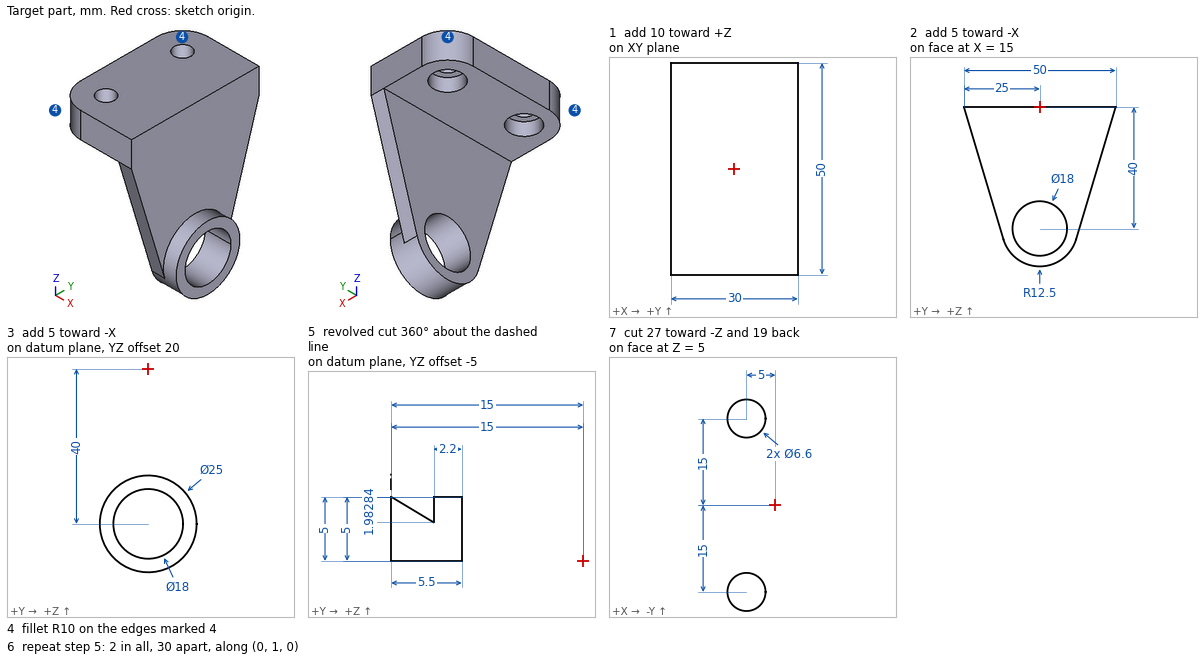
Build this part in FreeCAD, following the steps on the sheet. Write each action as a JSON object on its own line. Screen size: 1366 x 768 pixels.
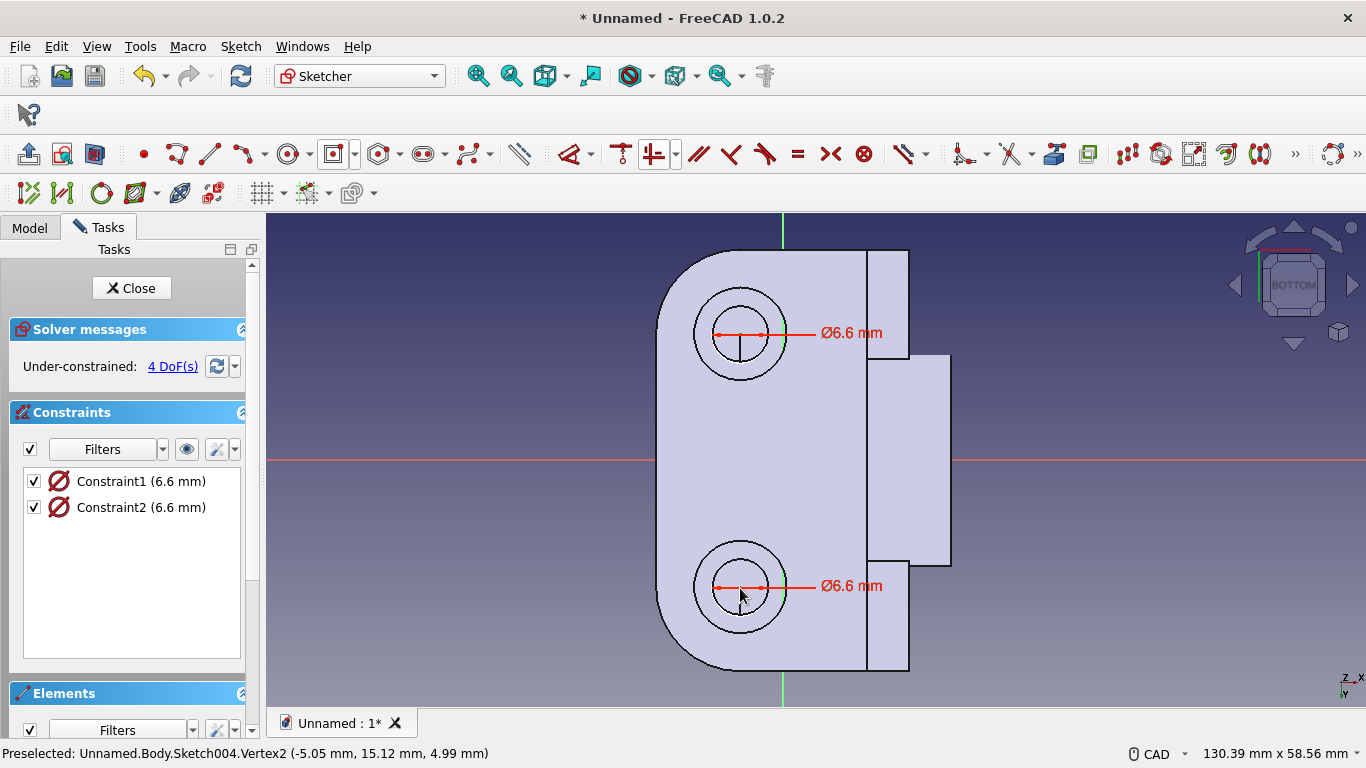
{"action": "key", "text": "v"}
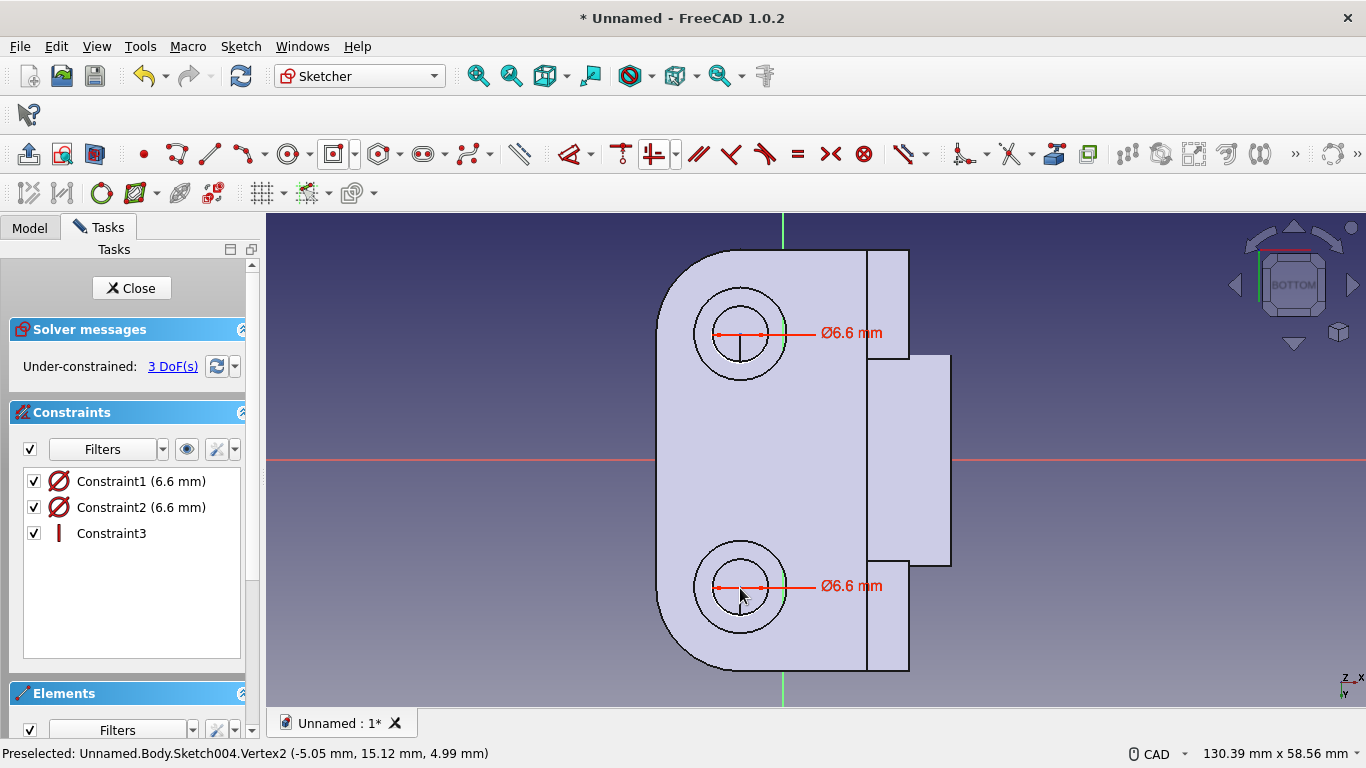
{"action": "left_click", "coordinate": [568, 154]}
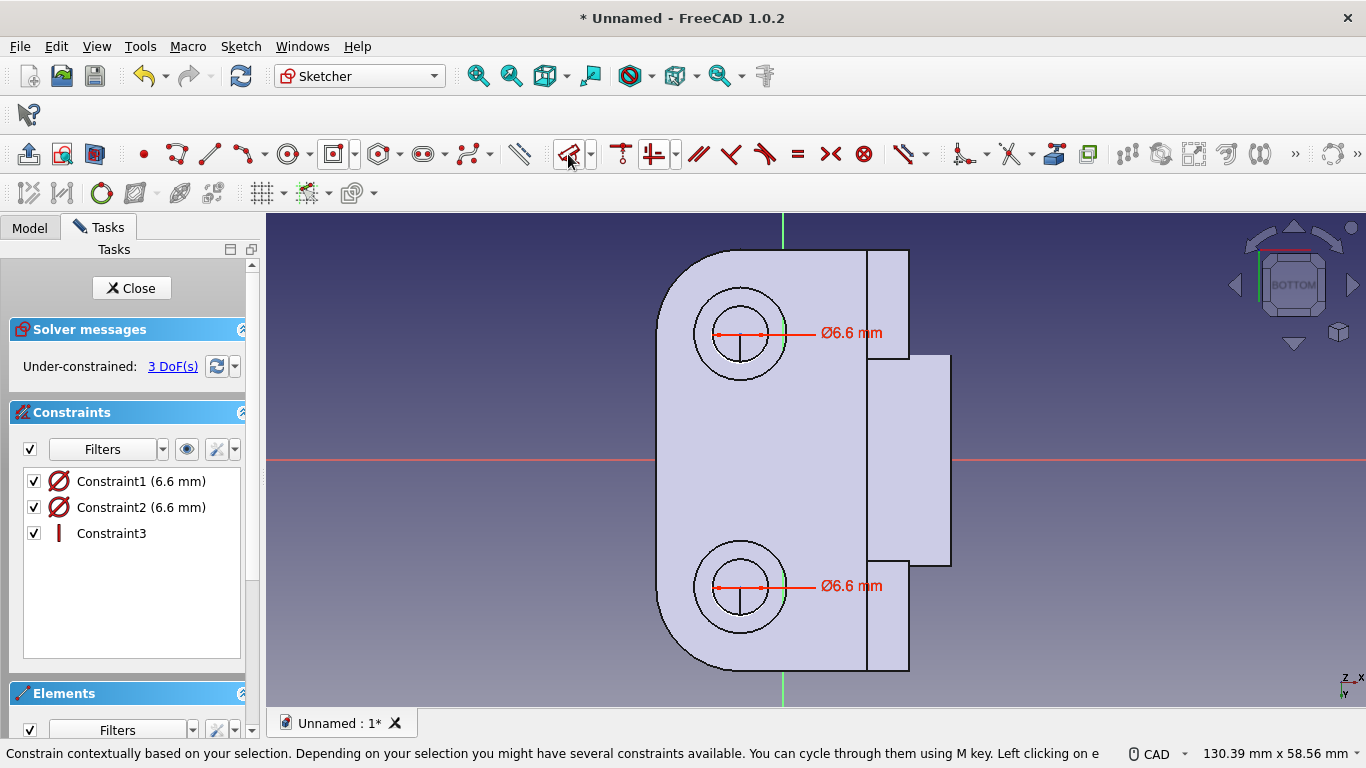
{"action": "left_click", "coordinate": [740, 335]}
{"action": "left_click", "coordinate": [761, 494]}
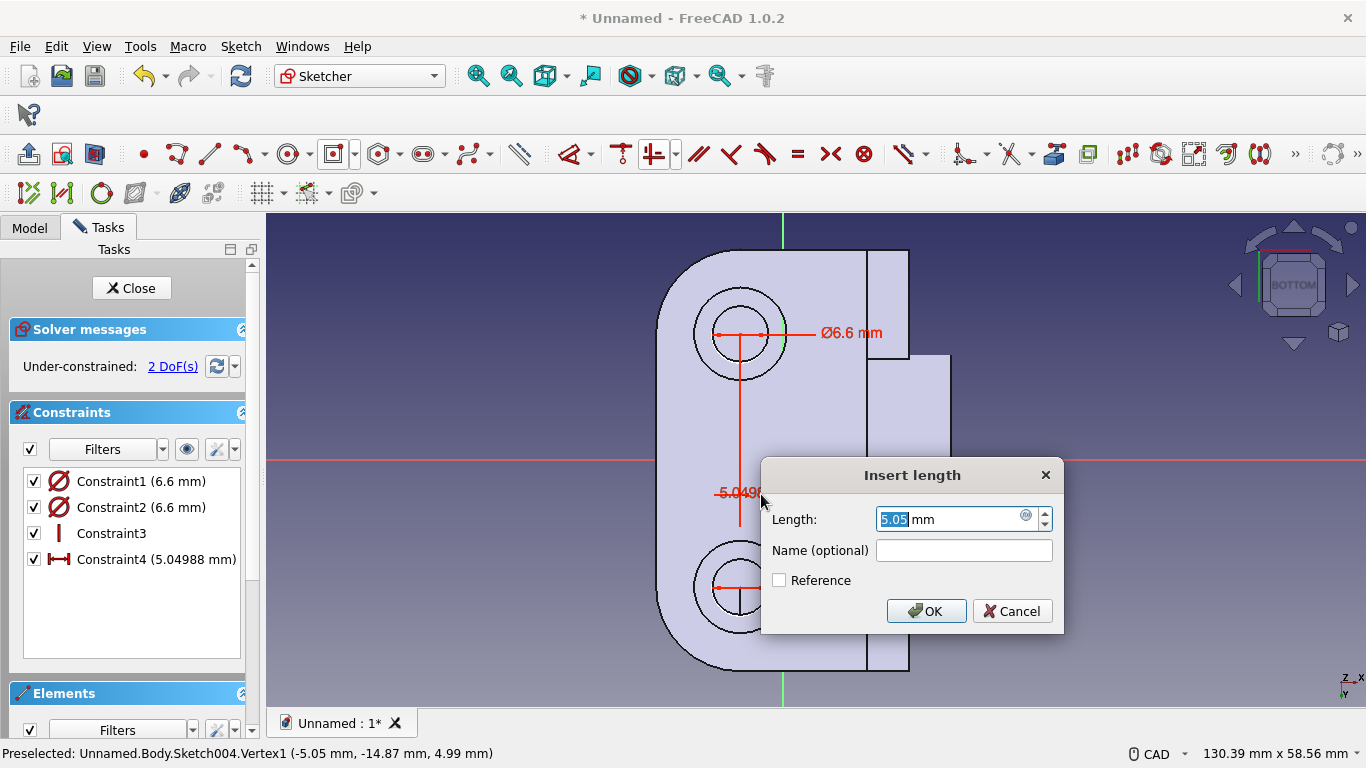
{"action": "type", "text": "5"}
{"action": "key", "text": "Return"}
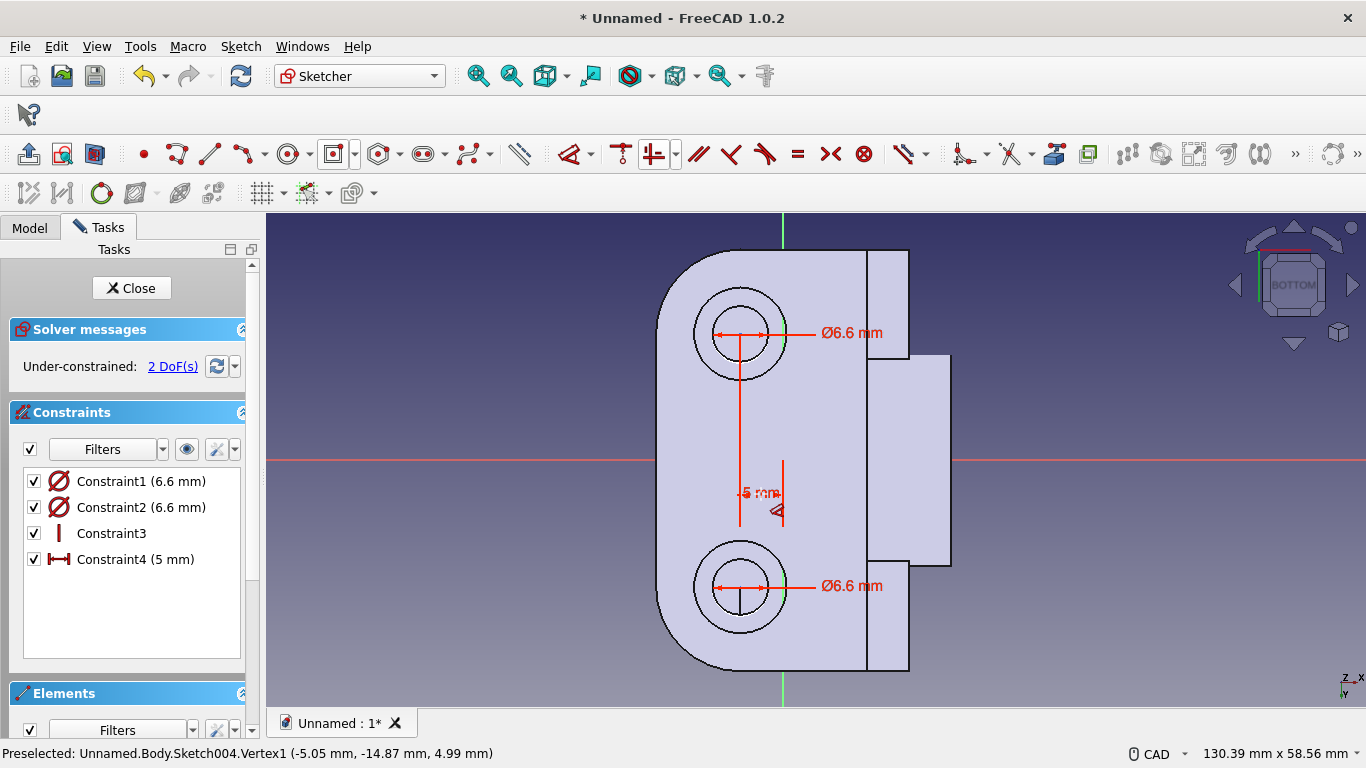
{"action": "left_click", "coordinate": [740, 335]}
{"action": "left_click", "coordinate": [817, 398]}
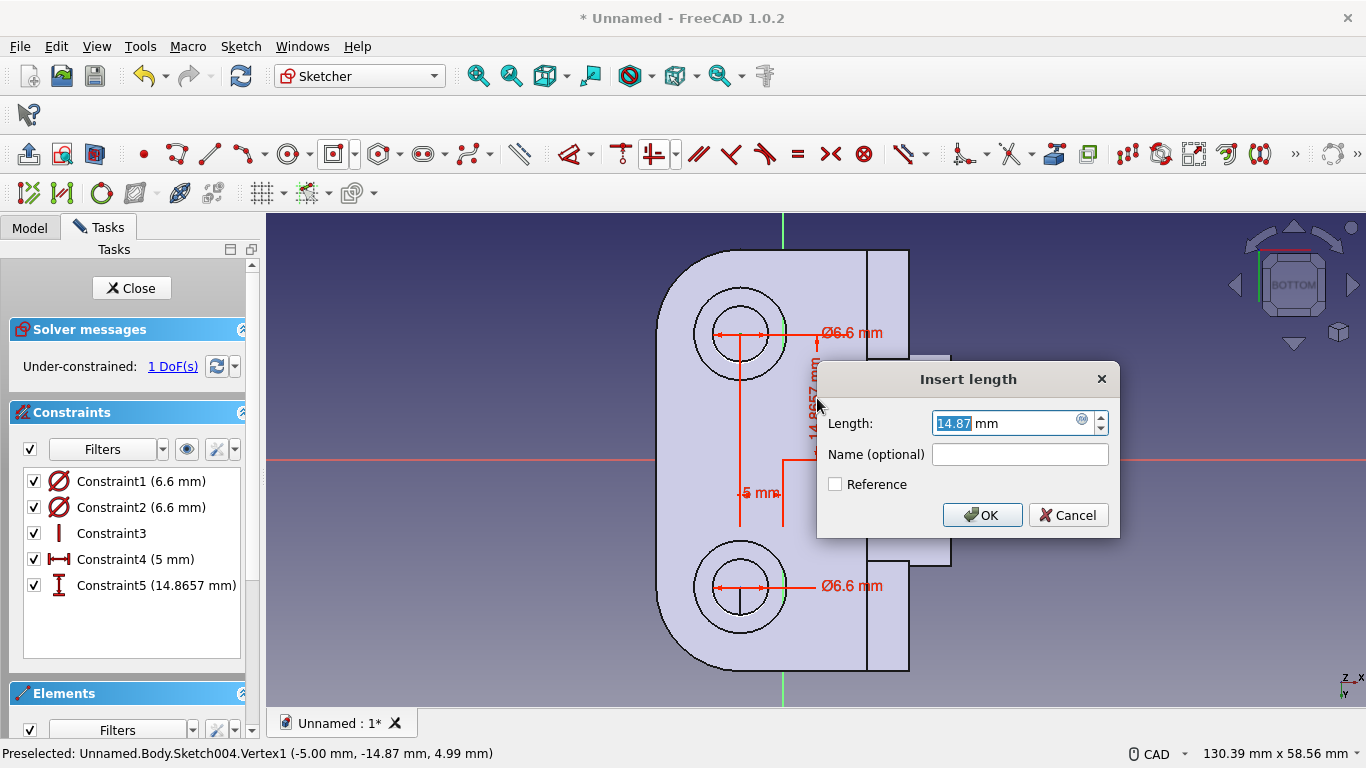
{"action": "type", "text": "15"}
{"action": "key", "text": "Return"}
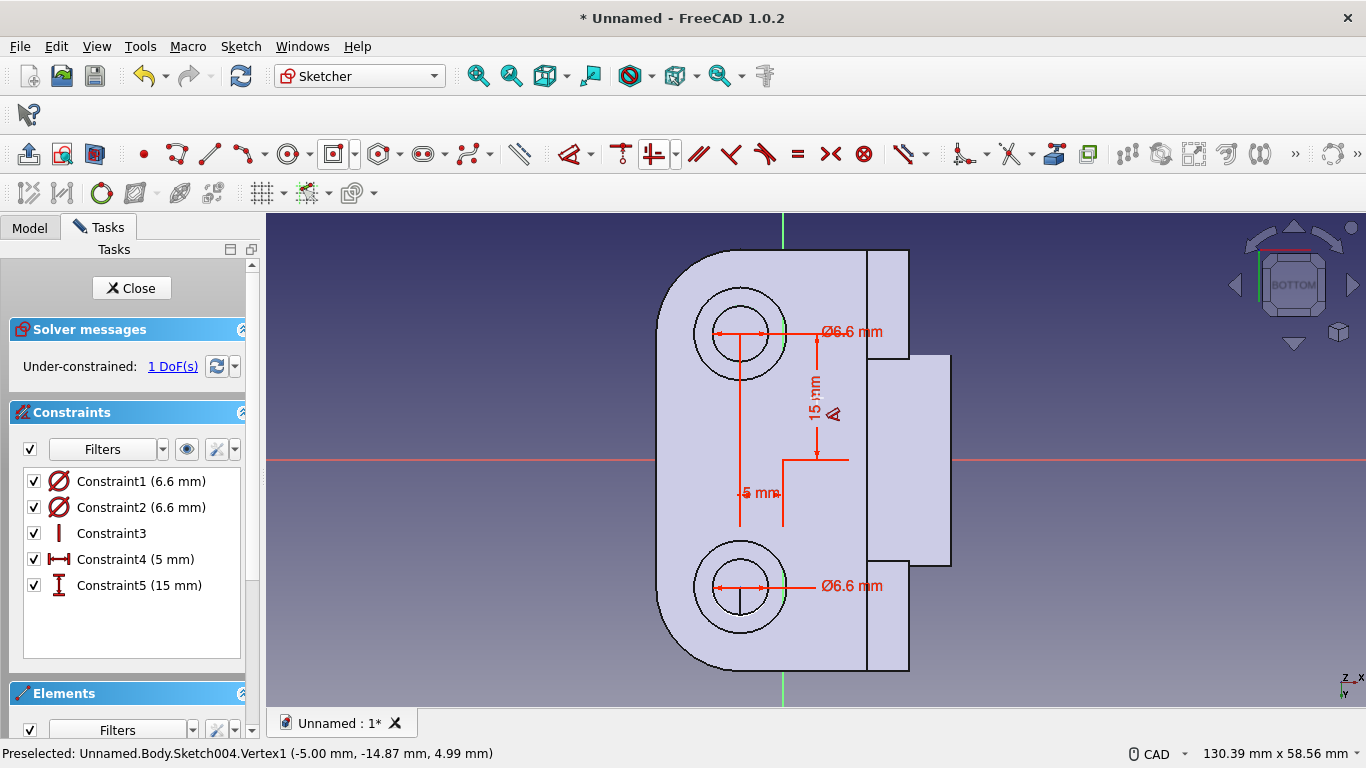
{"action": "left_click", "coordinate": [740, 588]}
{"action": "left_click", "coordinate": [817, 524]}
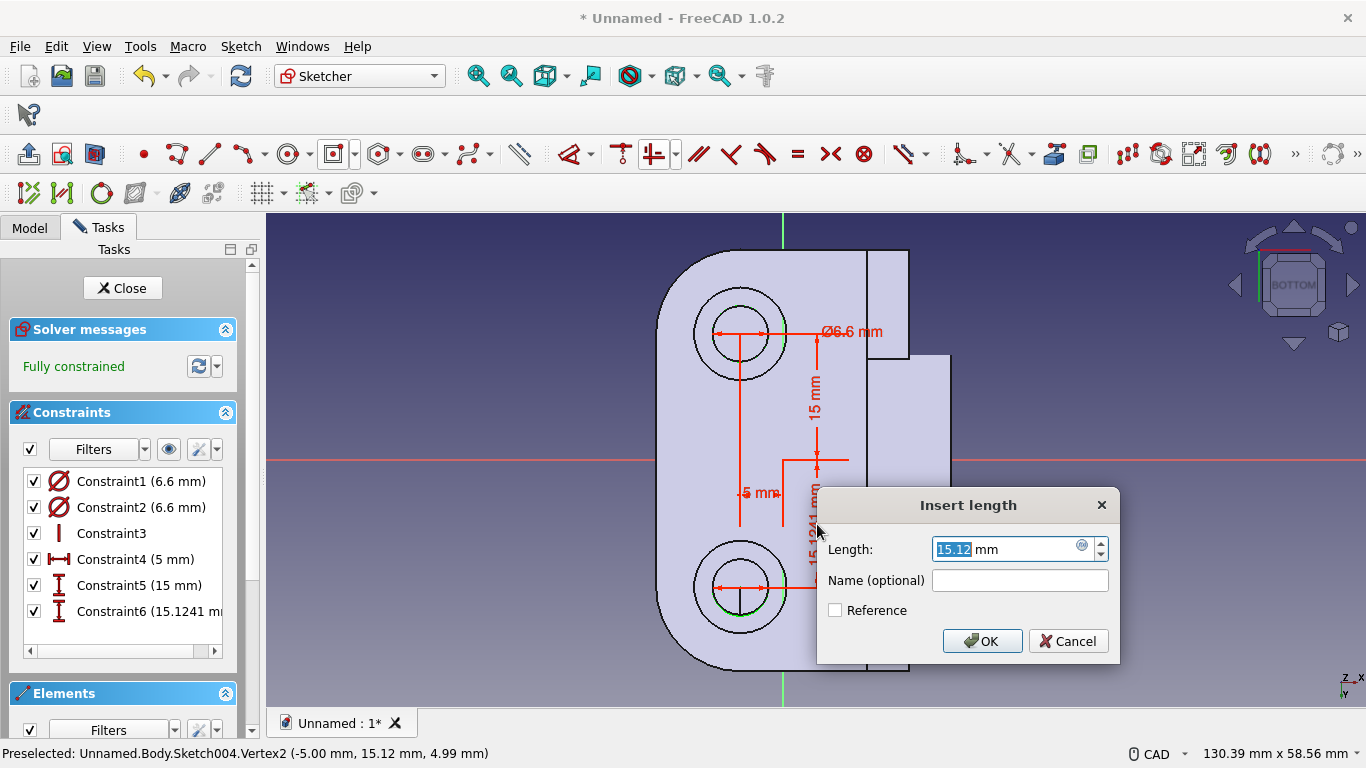
{"action": "type", "text": "15"}
{"action": "key", "text": "Return"}
{"action": "key", "text": "Escape"}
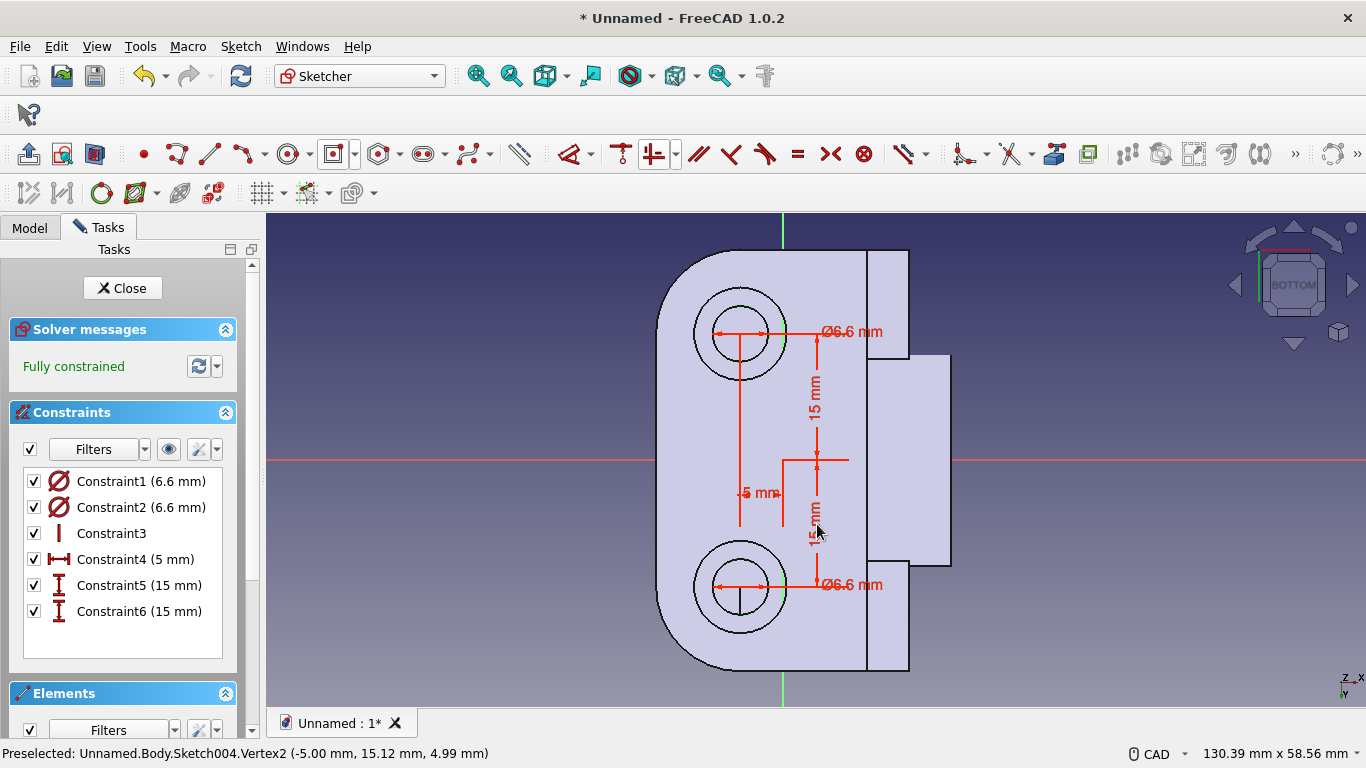
{"action": "left_click", "coordinate": [123, 288]}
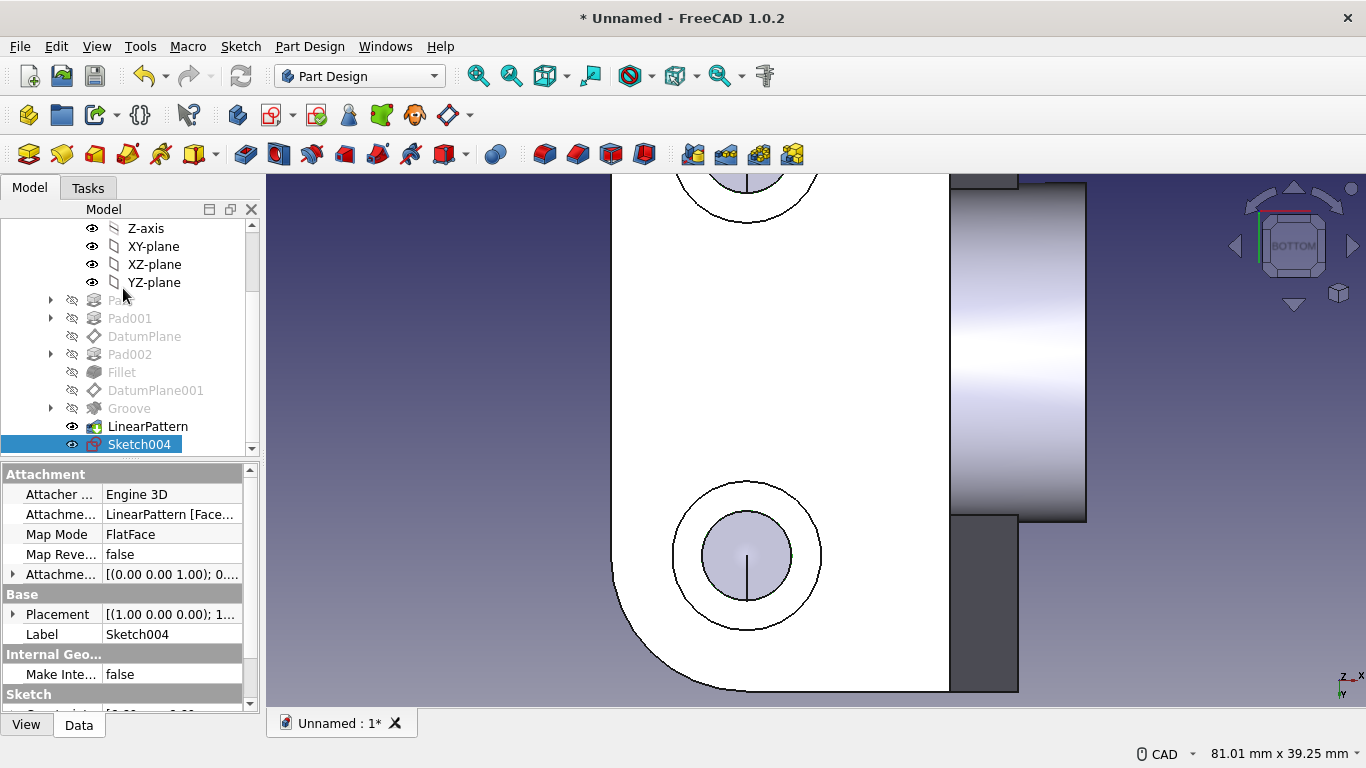
{"action": "left_click", "coordinate": [246, 154]}